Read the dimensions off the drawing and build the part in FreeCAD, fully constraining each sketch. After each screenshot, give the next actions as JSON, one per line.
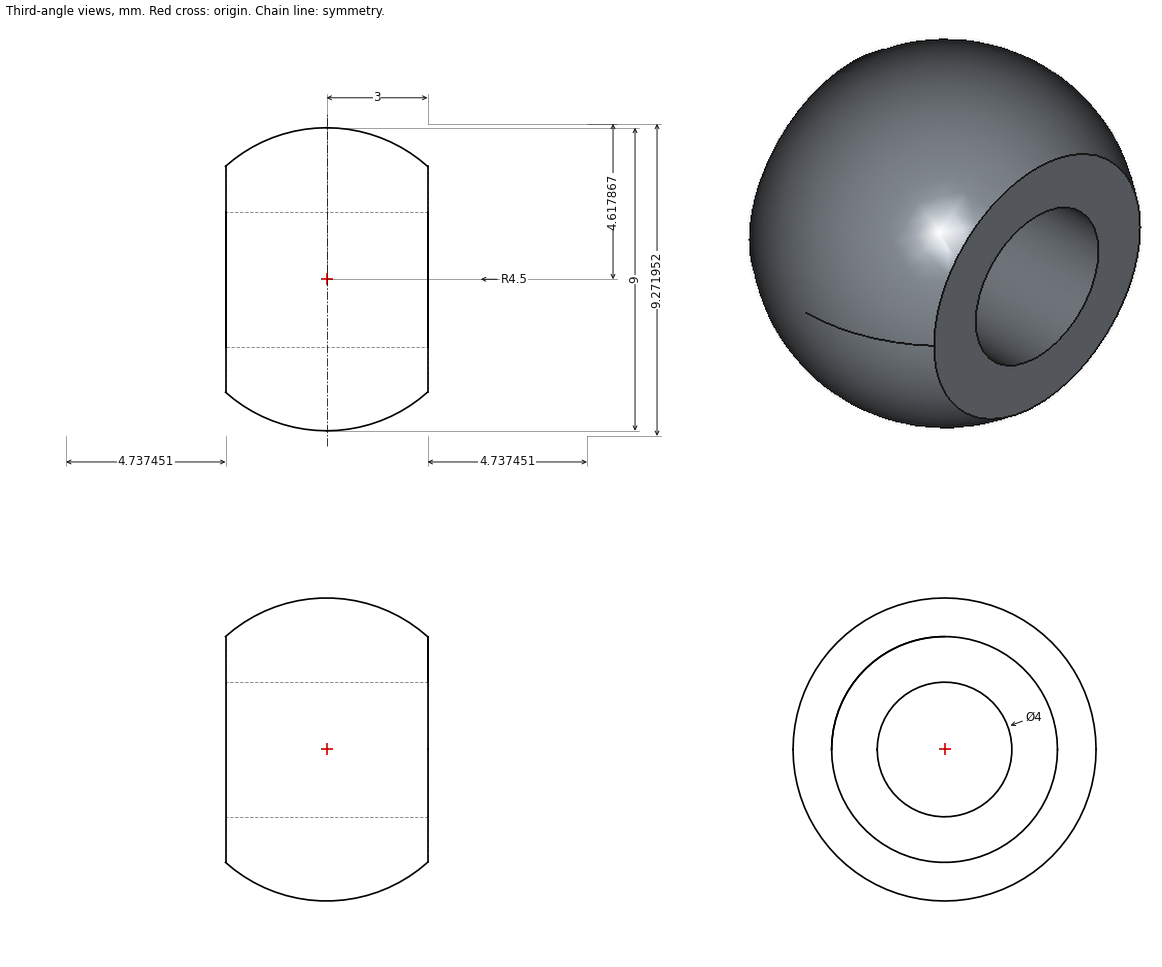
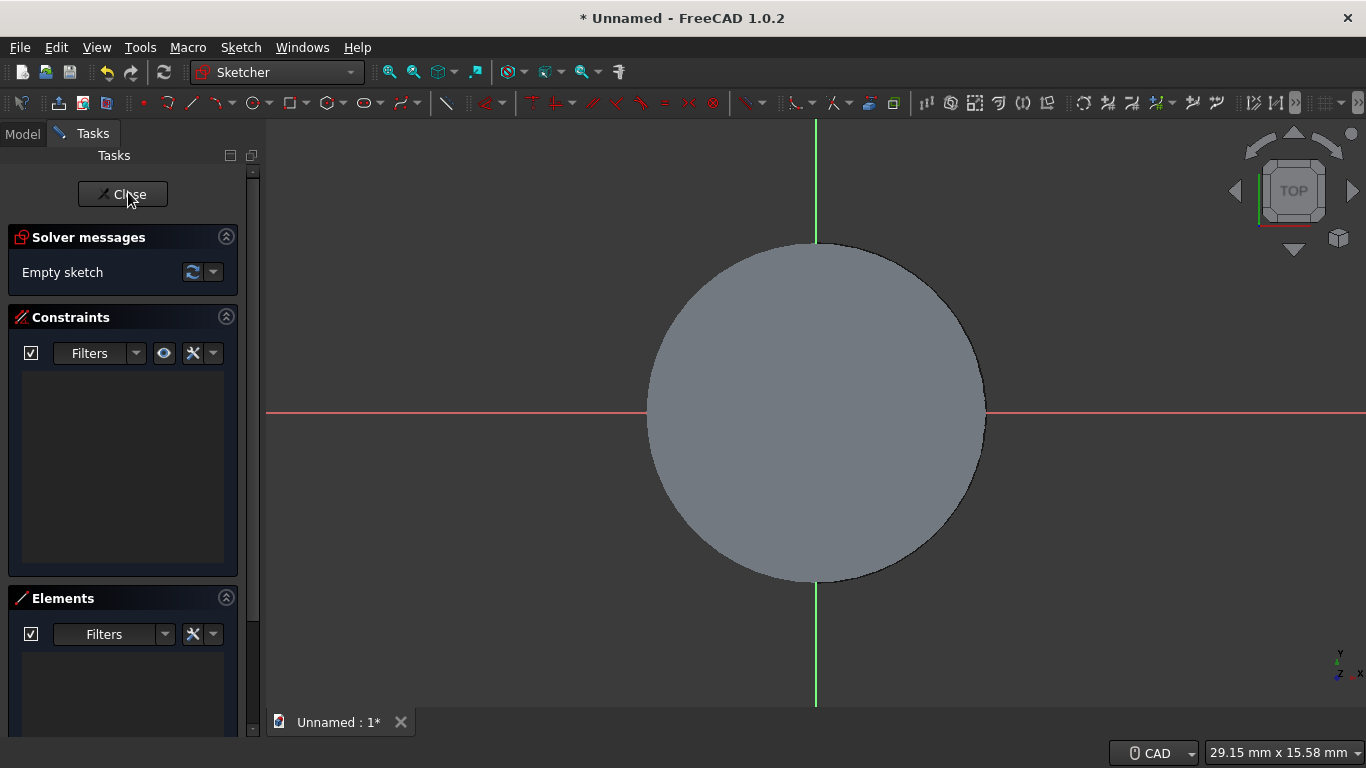
{"action": "key", "text": "q s"}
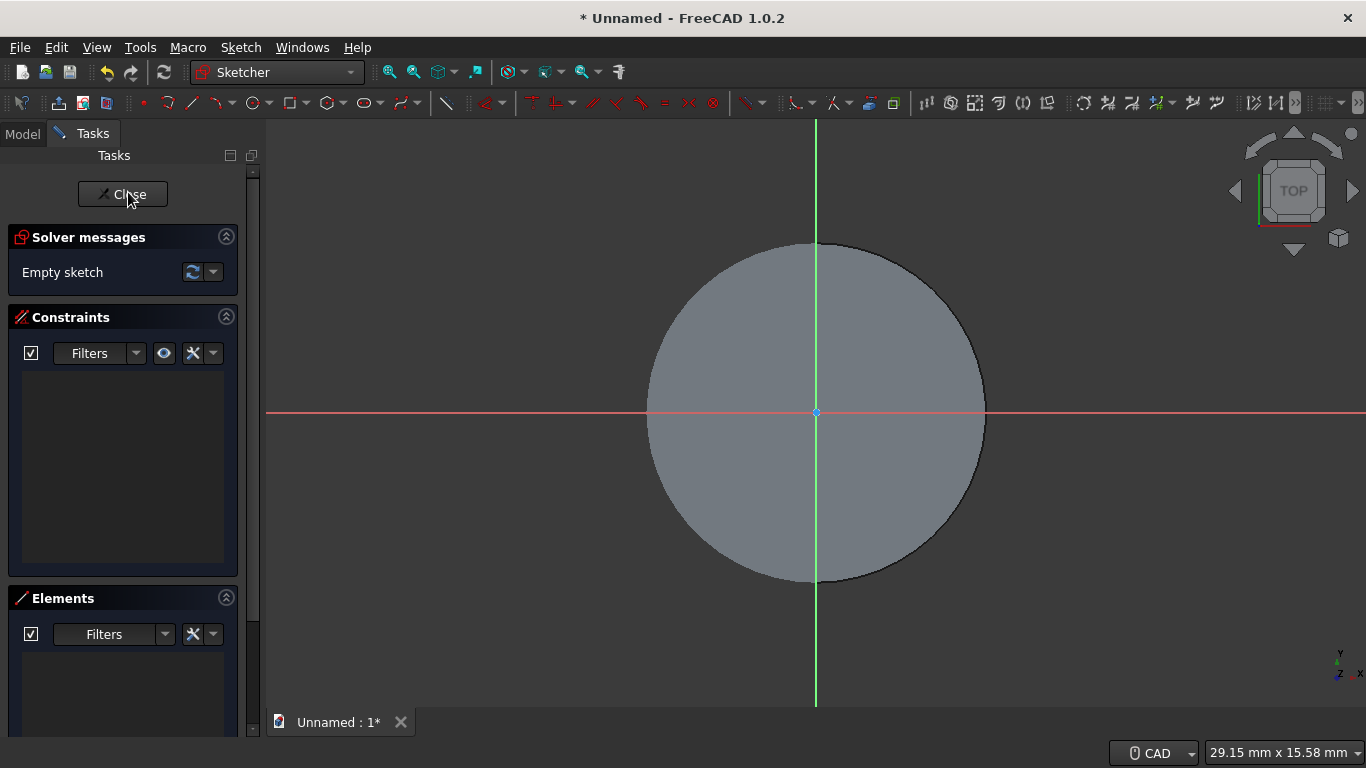
{"action": "key", "text": "g r"}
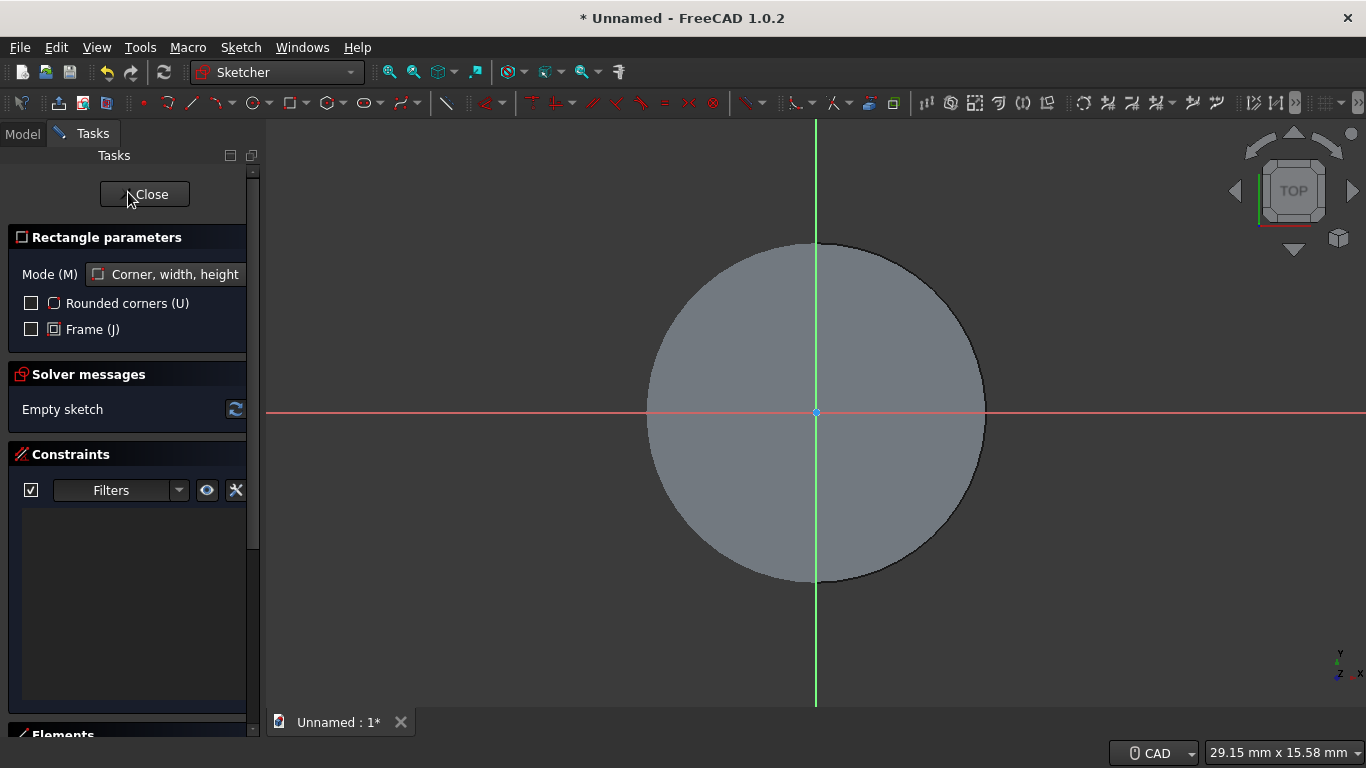
{"action": "left_click", "coordinate": [929, 239]}
{"action": "mouse_move", "coordinate": [1108, 589]}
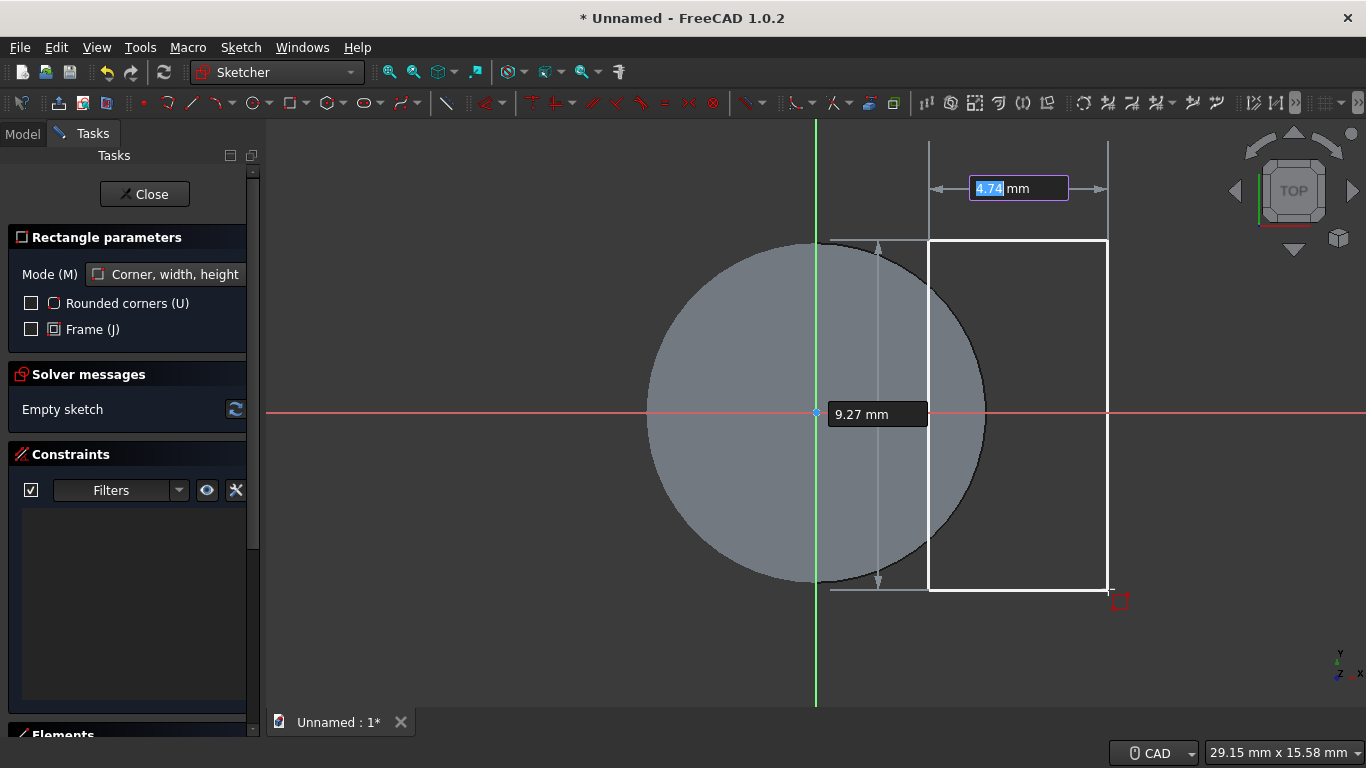
{"action": "type", "text": "4.737451"}
{"action": "key", "text": "Tab"}
{"action": "type", "text": "9.271952"}
{"action": "key", "text": "Return"}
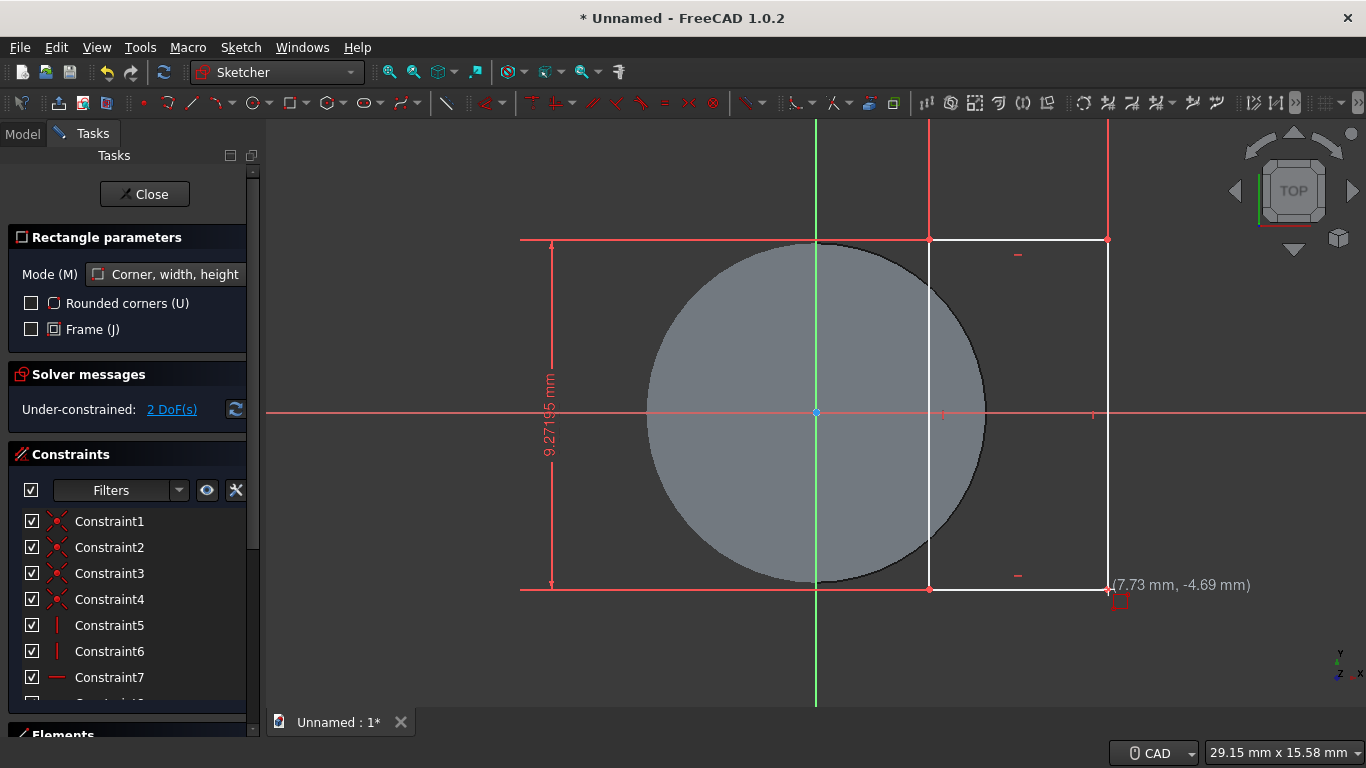
{"action": "left_click", "coordinate": [524, 239]}
{"action": "mouse_move", "coordinate": [703, 589]}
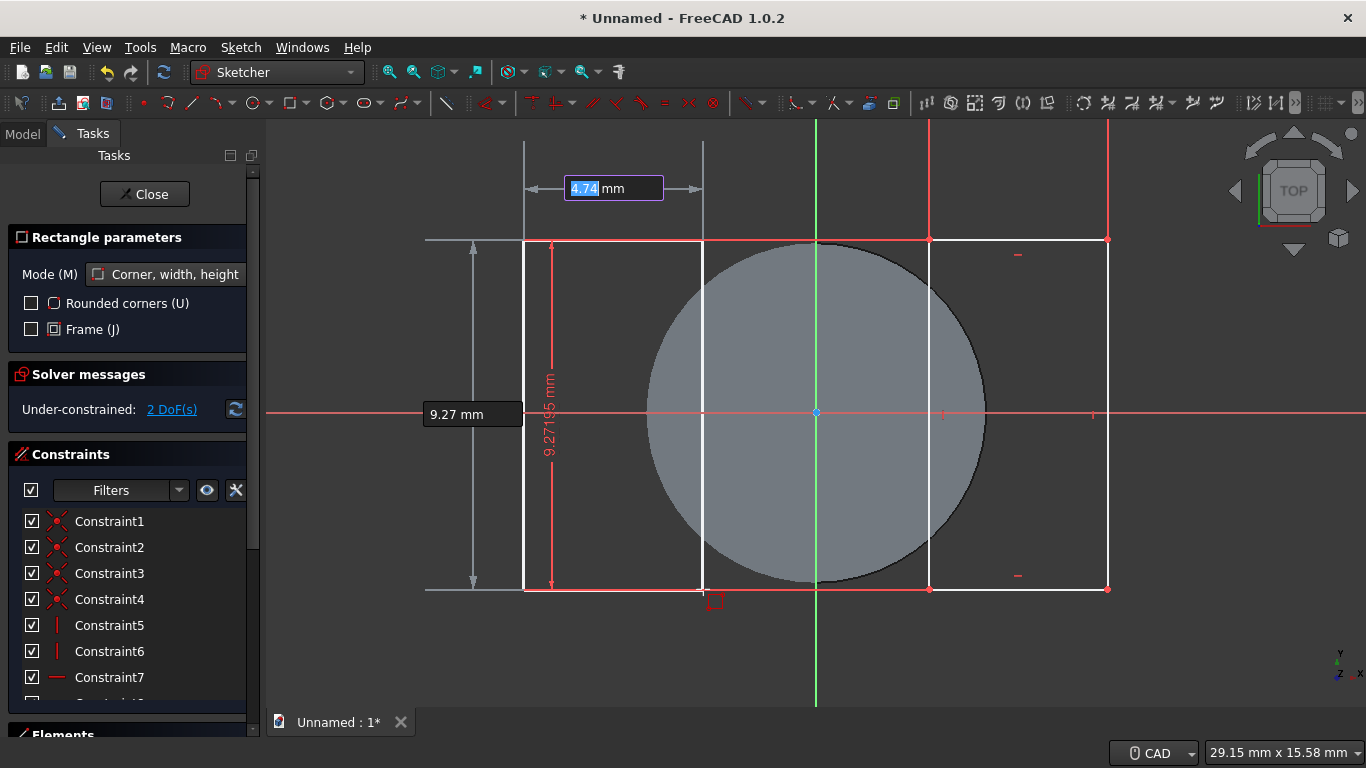
{"action": "type", "text": "4.737451"}
{"action": "key", "text": "Tab"}
{"action": "type", "text": "9.271952"}
{"action": "key", "text": "Return"}
{"action": "key", "text": "Escape"}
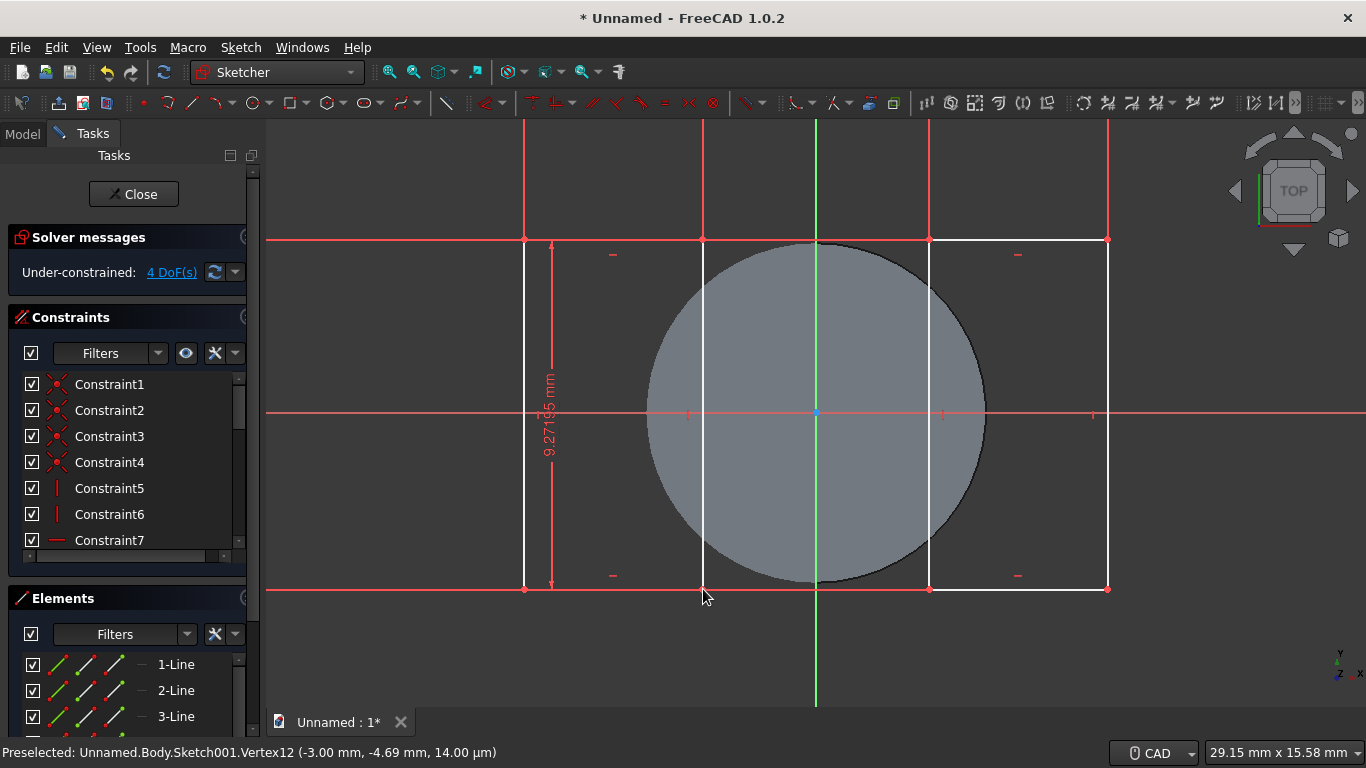
{"action": "left_click", "coordinate": [1108, 240]}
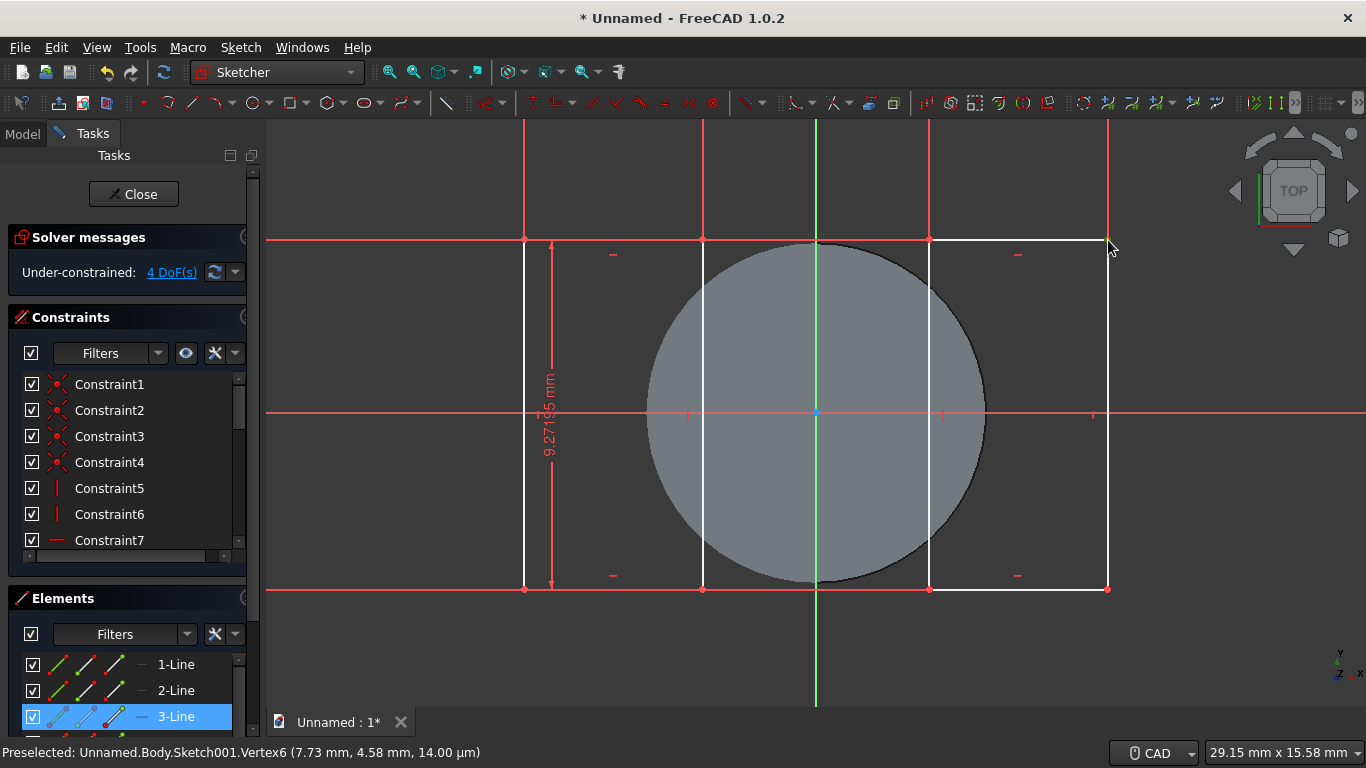
{"action": "left_click", "coordinate": [524, 240]}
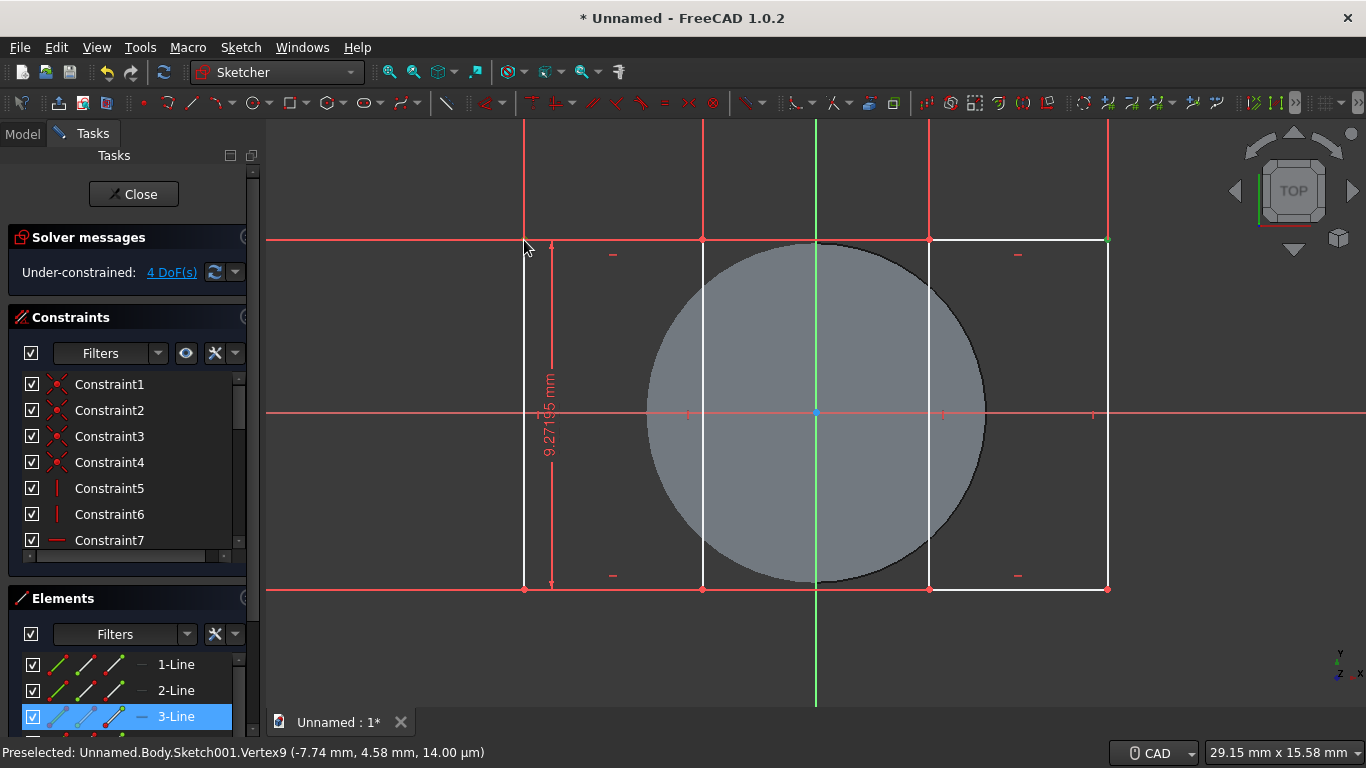
{"action": "left_click", "coordinate": [816, 641]}